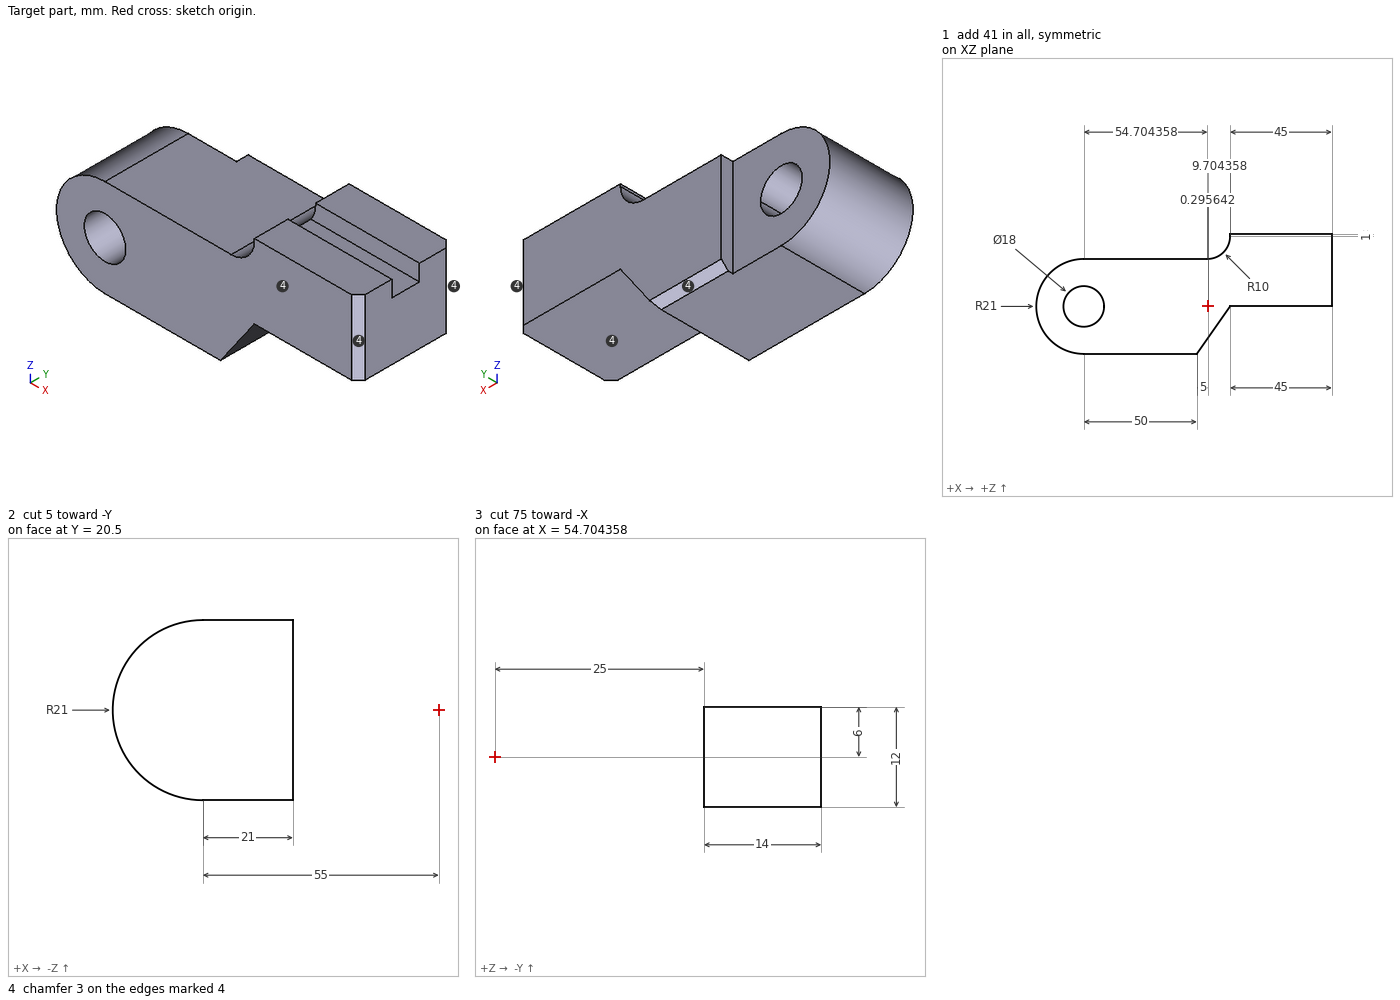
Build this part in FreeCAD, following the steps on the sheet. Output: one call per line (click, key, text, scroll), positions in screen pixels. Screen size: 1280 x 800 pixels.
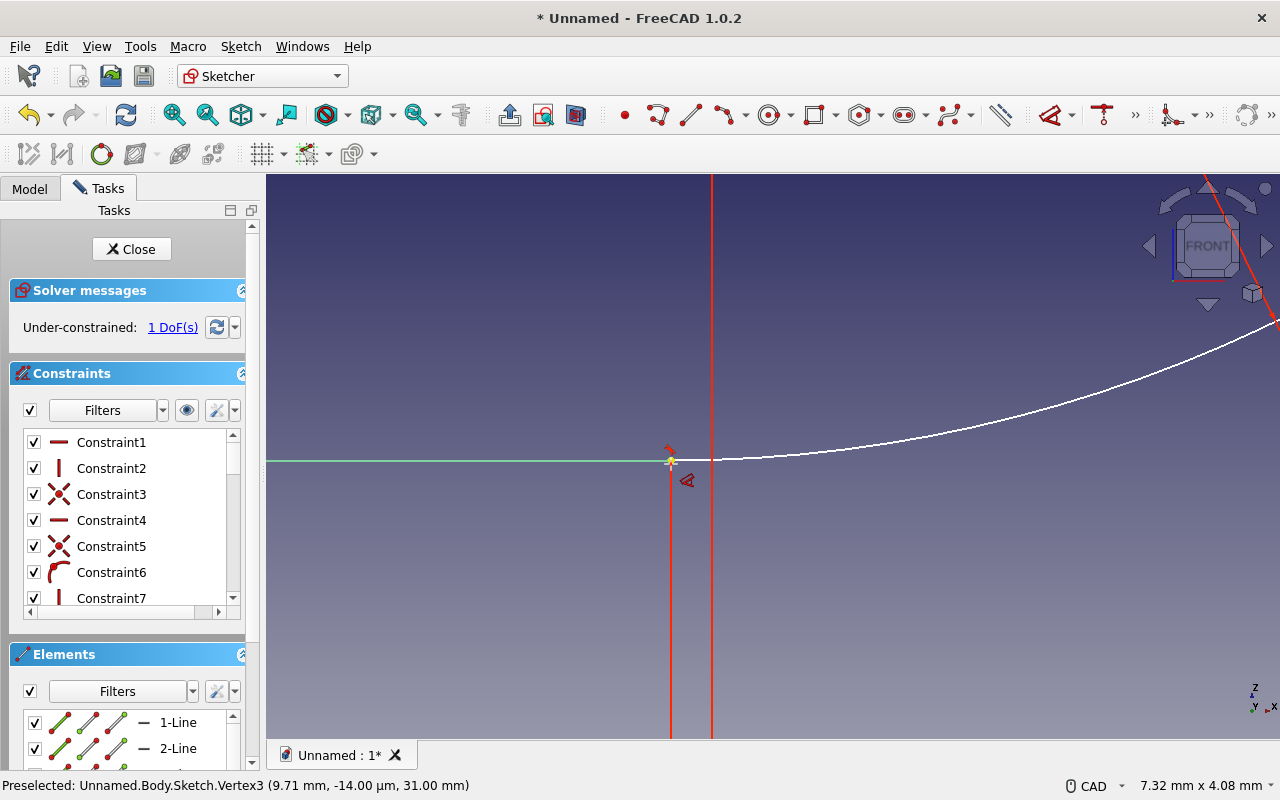
click(672, 461)
click(692, 427)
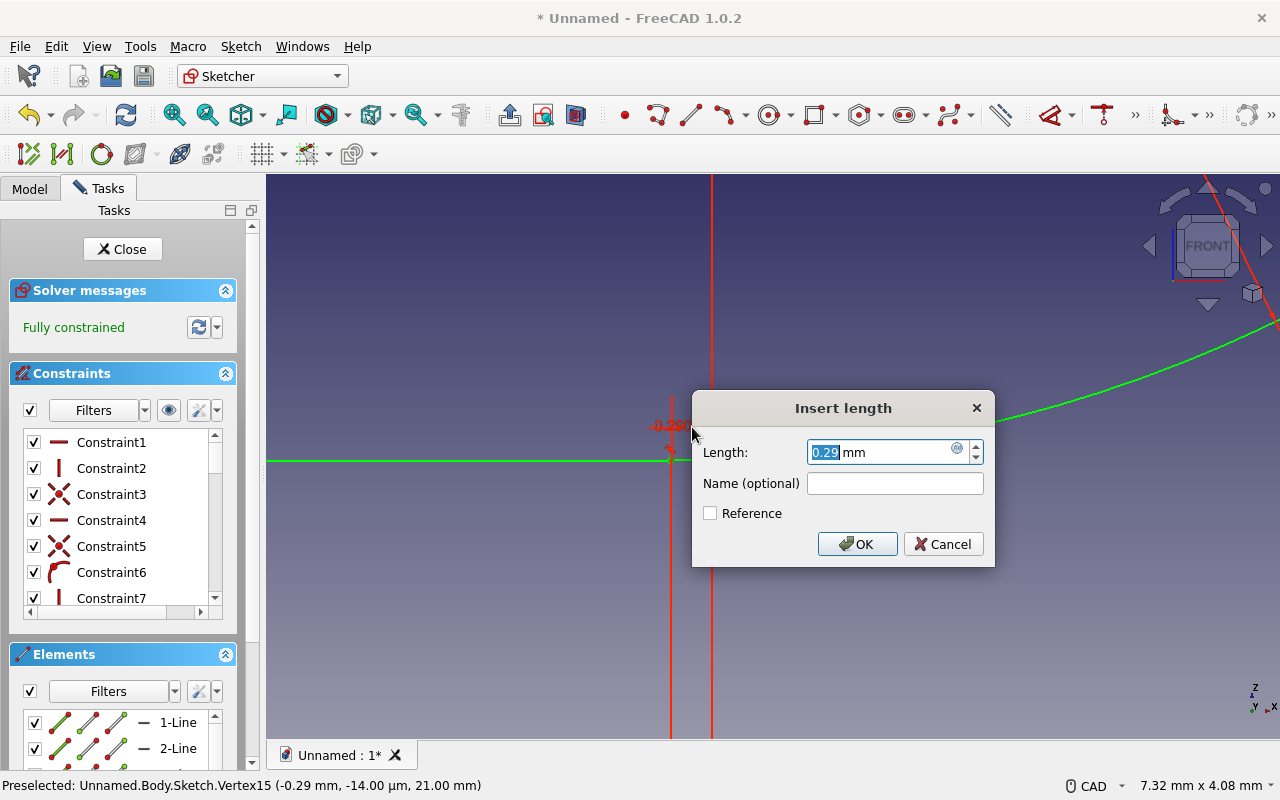
text(0.295642)
key(Return)
key(Escape)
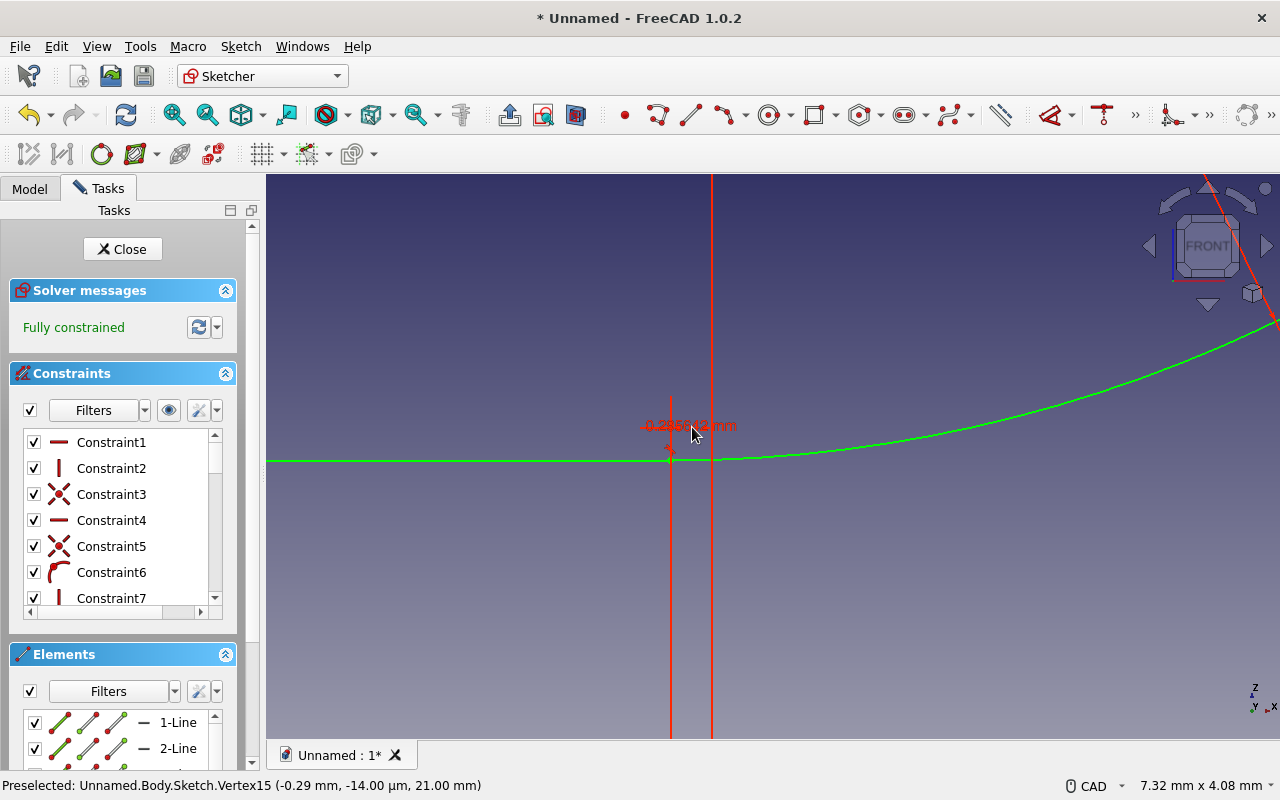
click(123, 249)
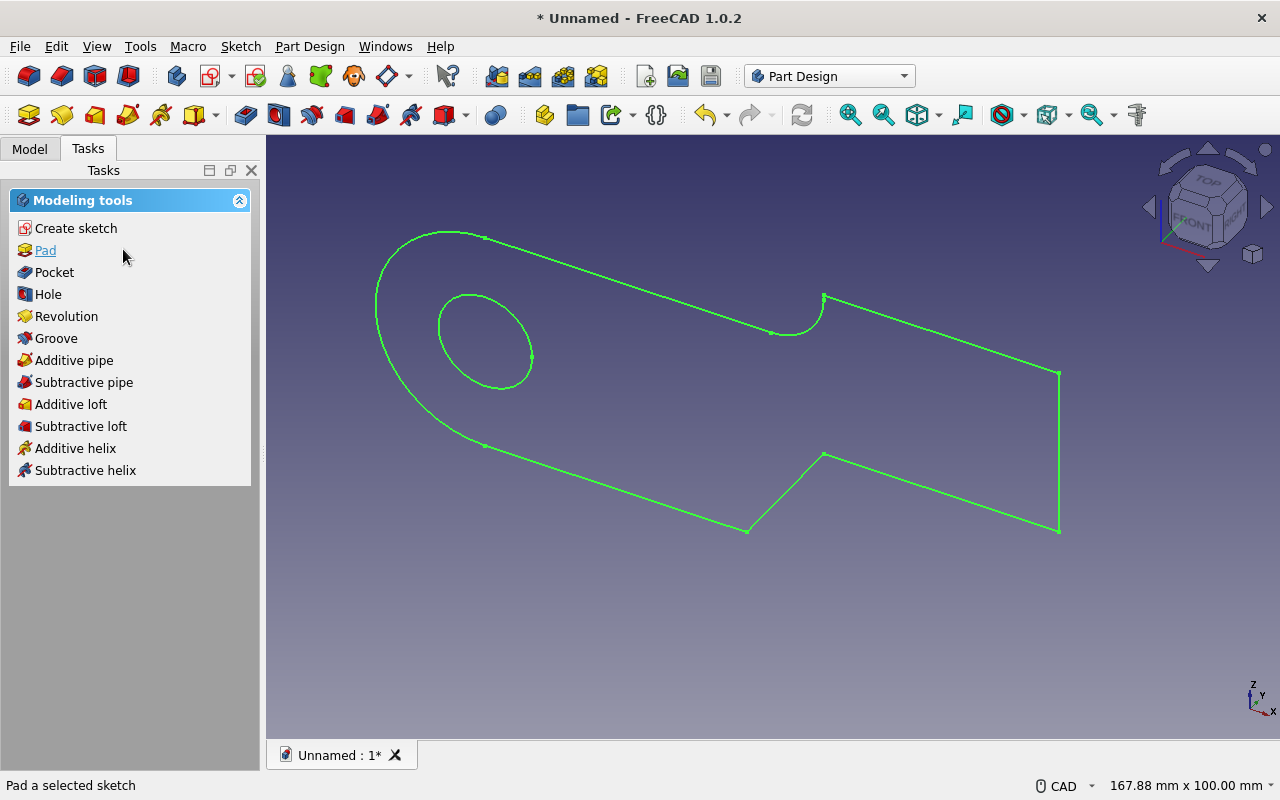
click(29, 116)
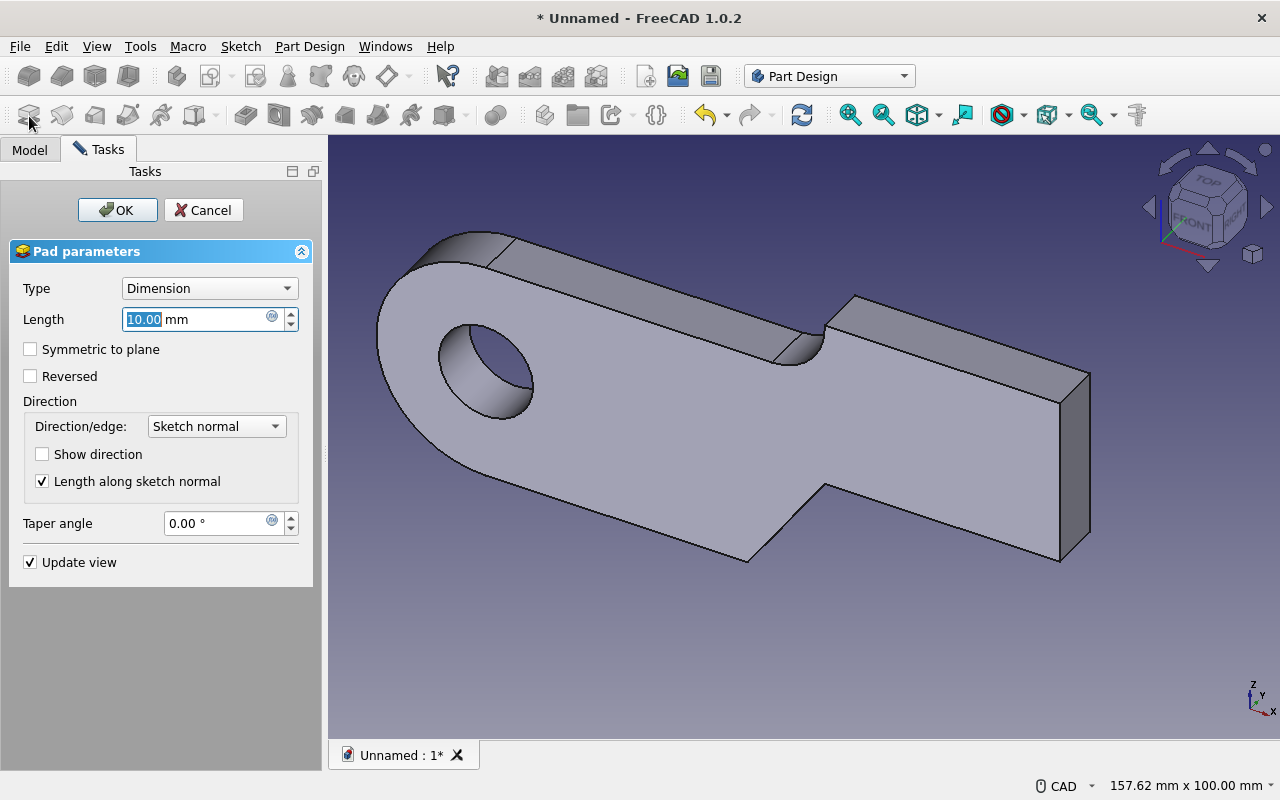
text(41)
key(Tab)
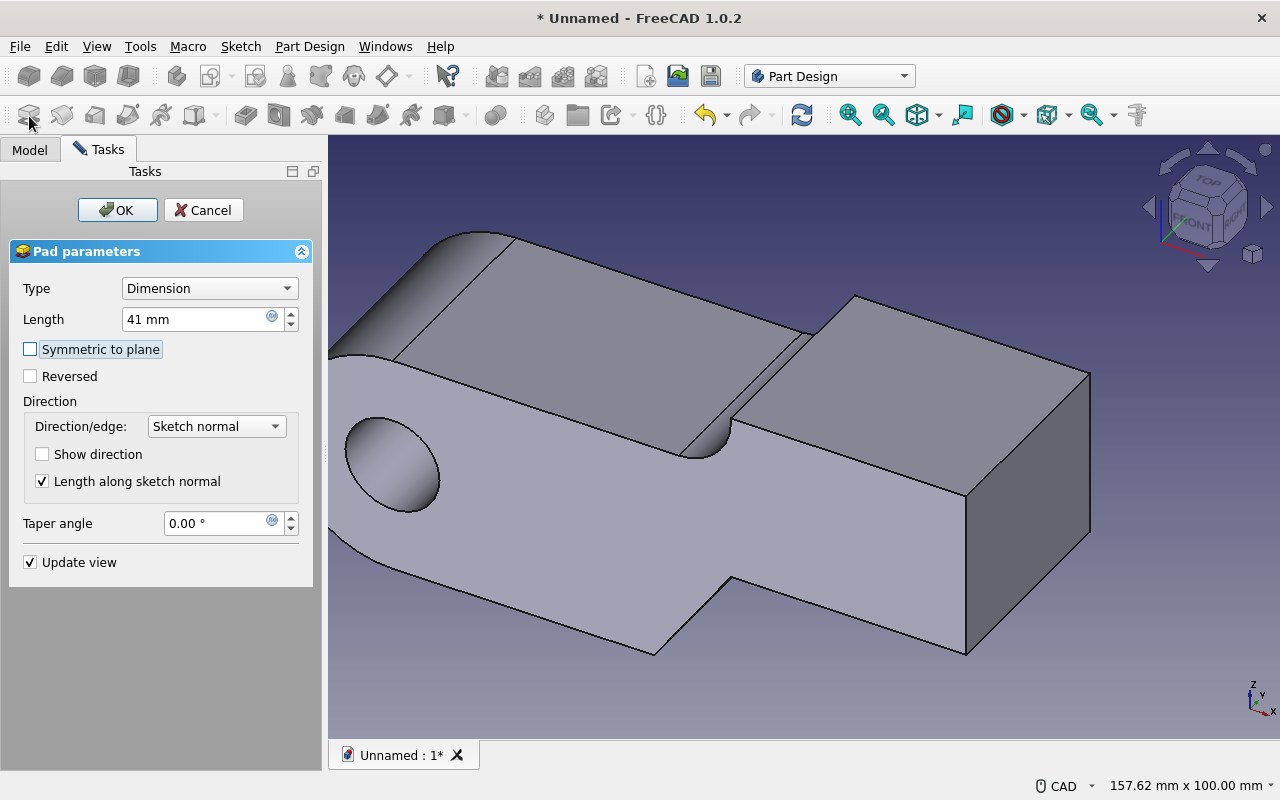
click(31, 349)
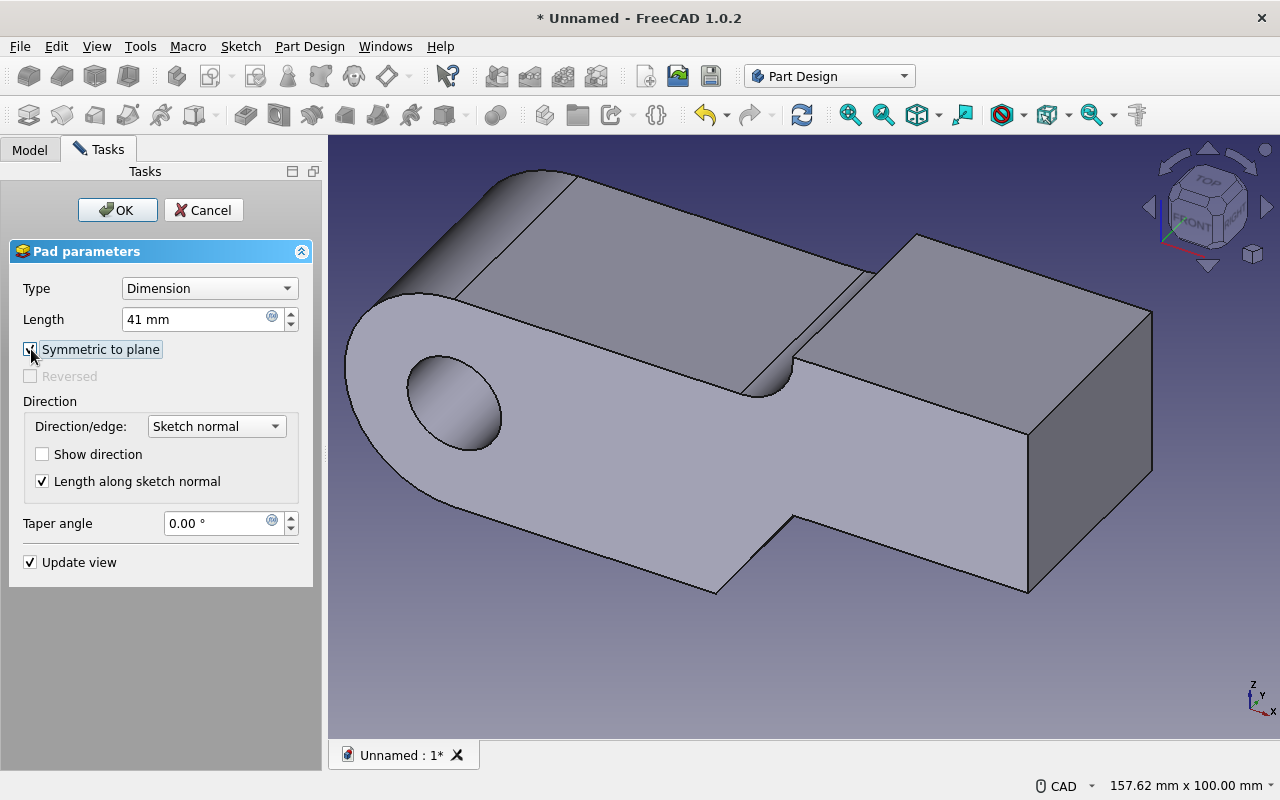
click(118, 210)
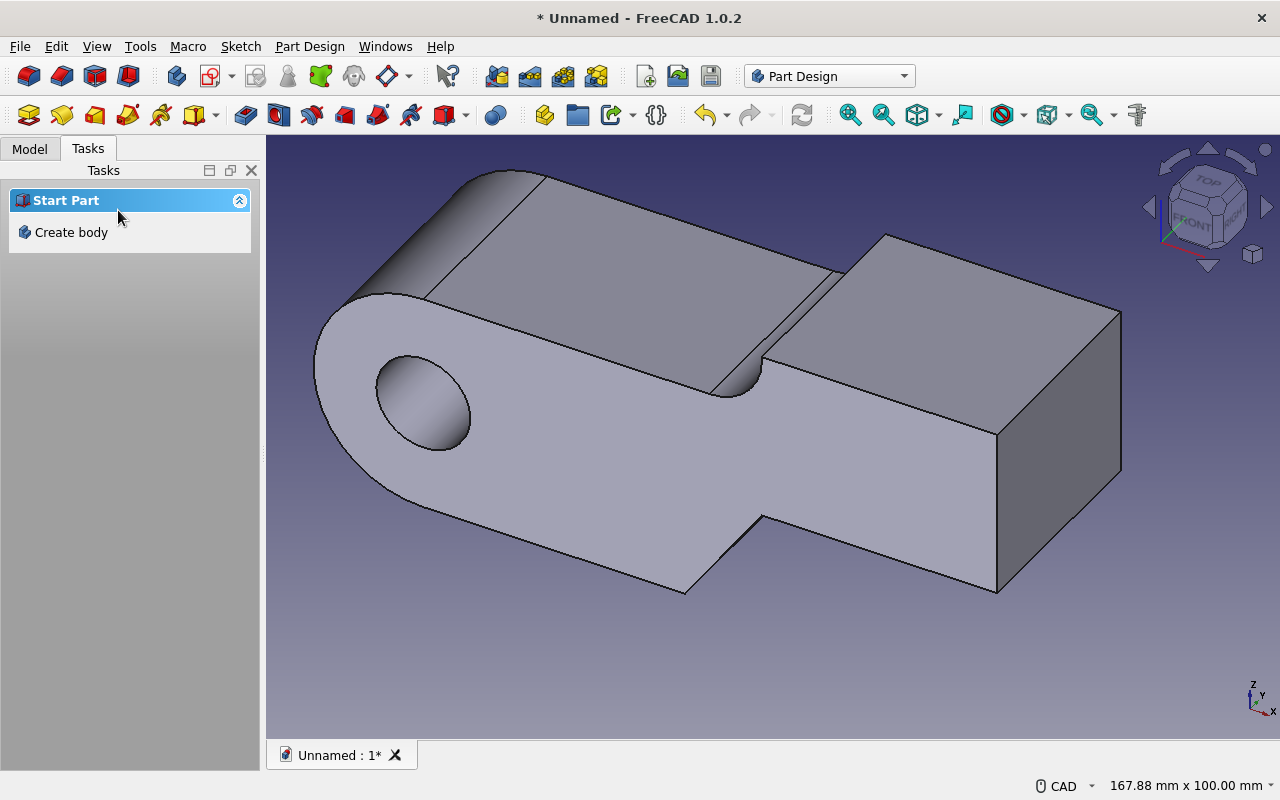
key(v)
key(f)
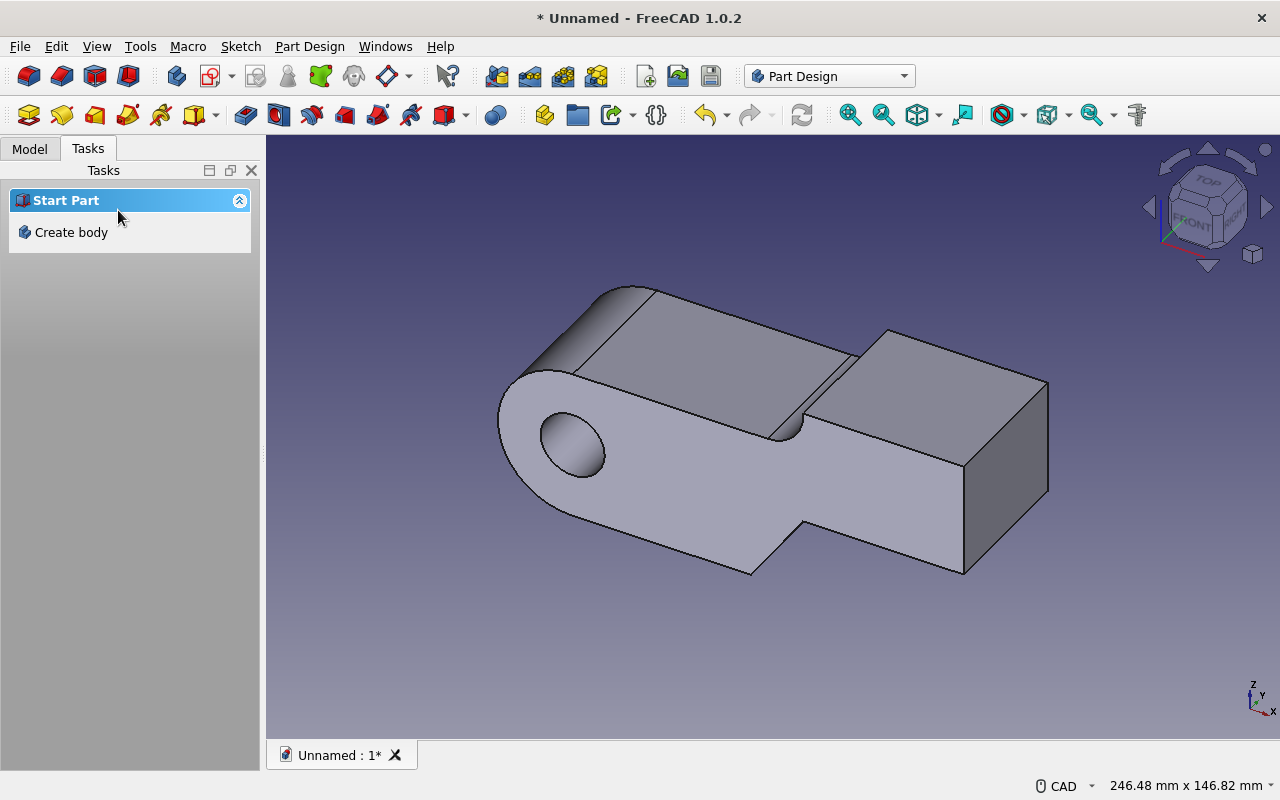
key(4)